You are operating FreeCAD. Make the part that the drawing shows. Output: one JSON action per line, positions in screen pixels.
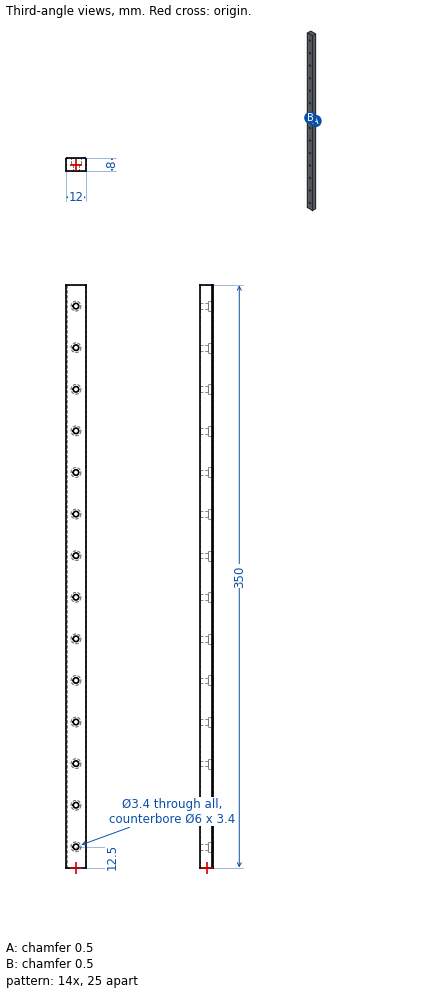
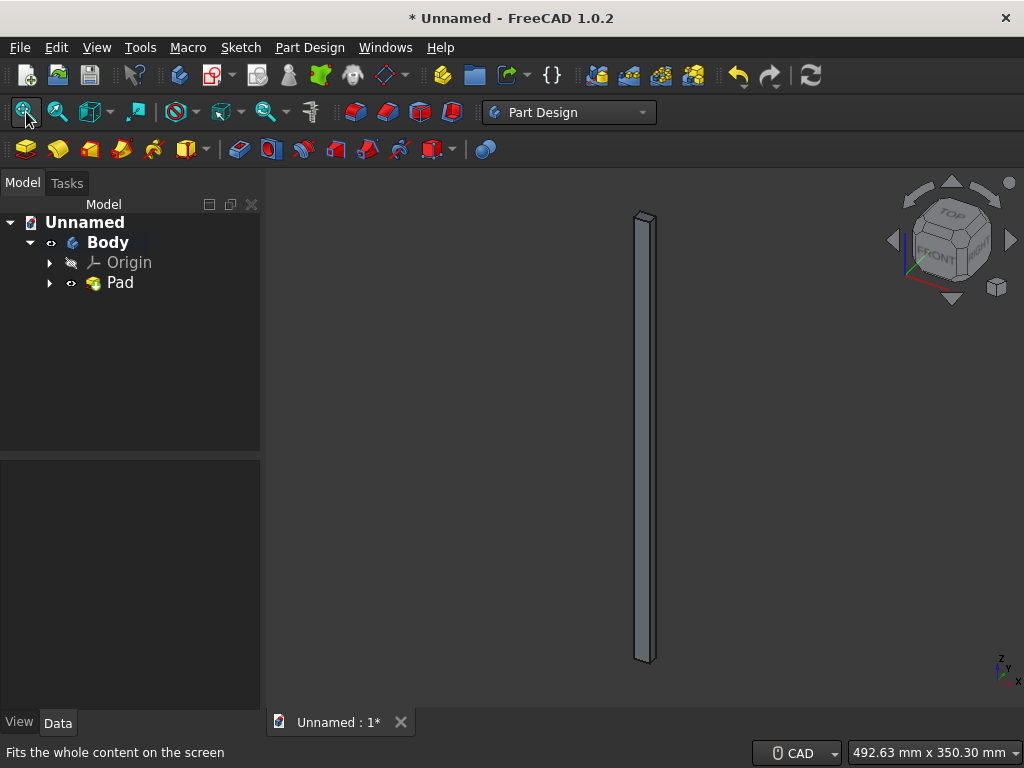
{"action": "key", "text": "0"}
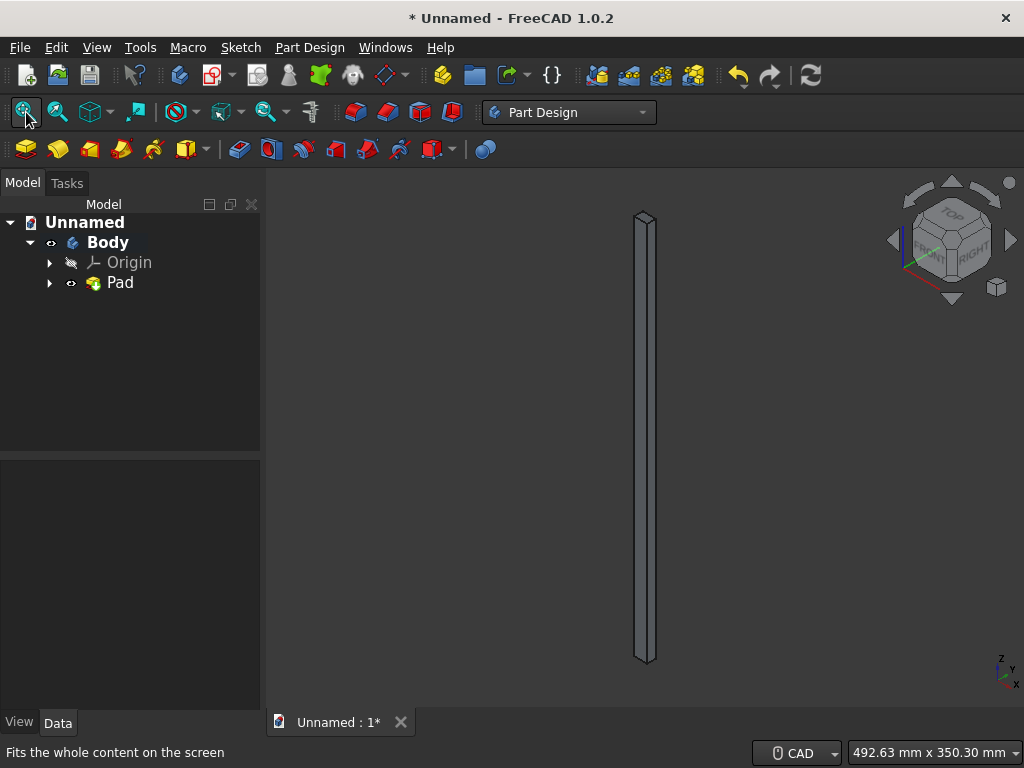
{"action": "key", "text": "2"}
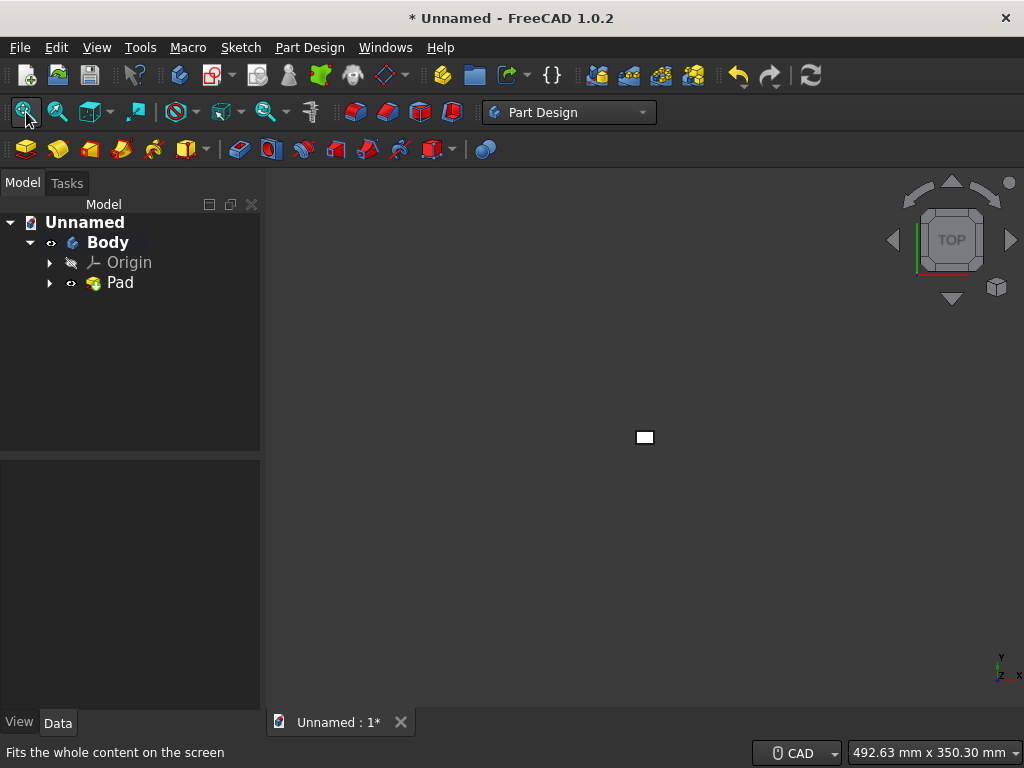
{"action": "left_click", "coordinate": [26, 112]}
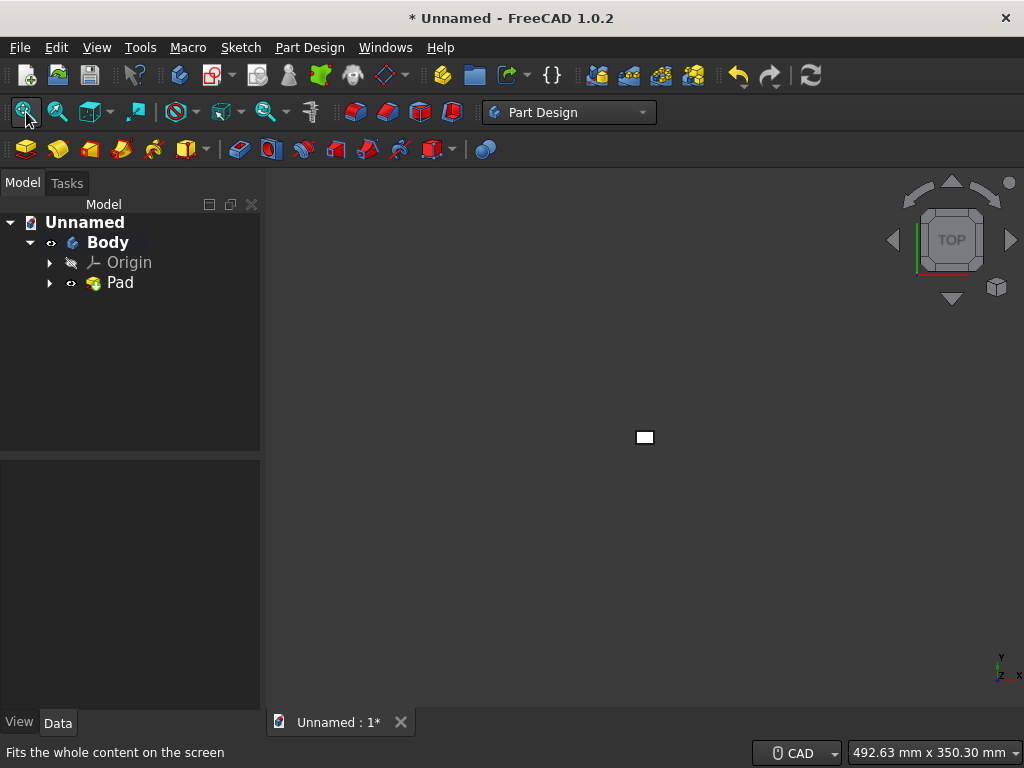
{"action": "key", "text": "1"}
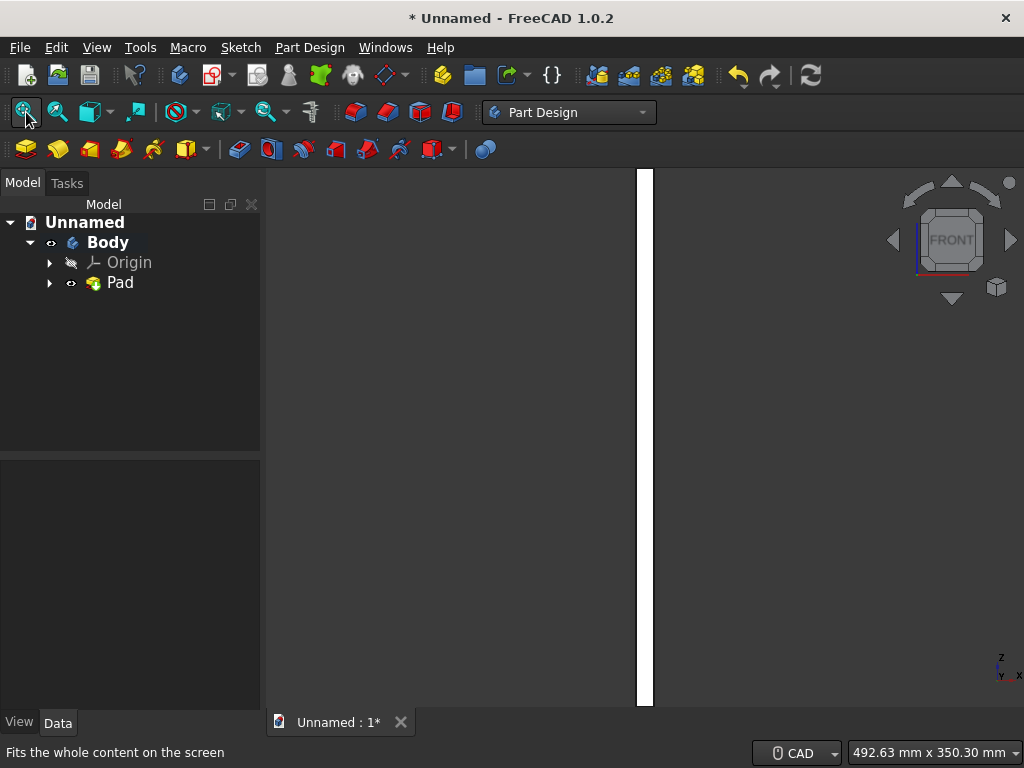
{"action": "left_click", "coordinate": [26, 112]}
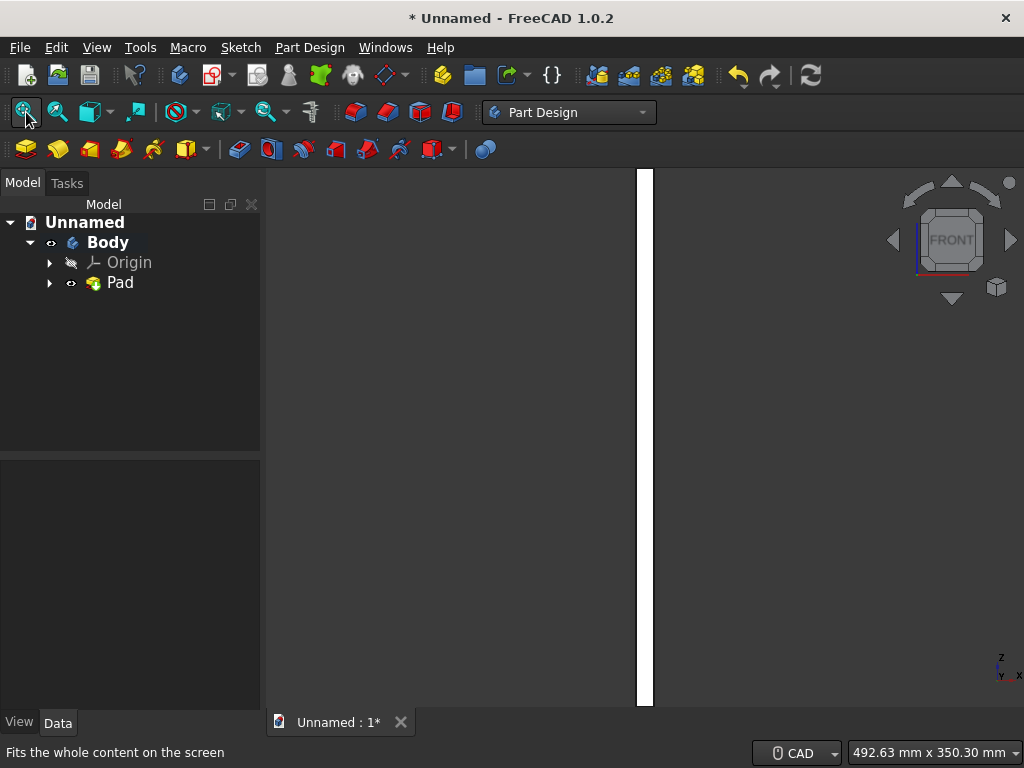
{"action": "key", "text": "3"}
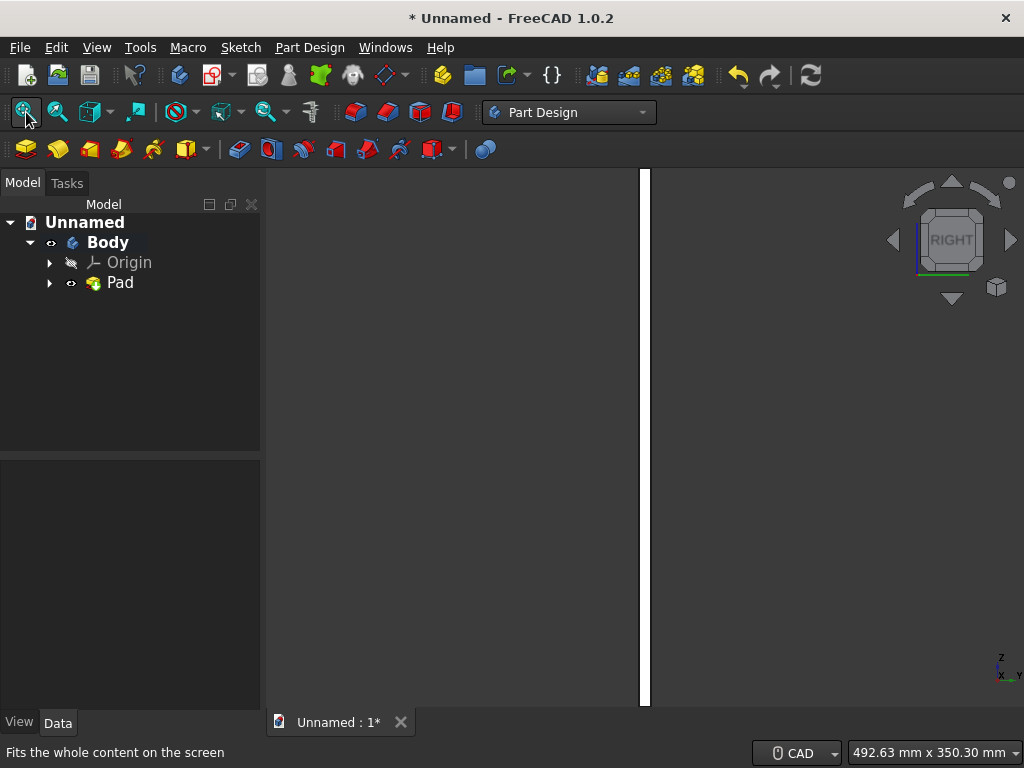
{"action": "left_click", "coordinate": [26, 112]}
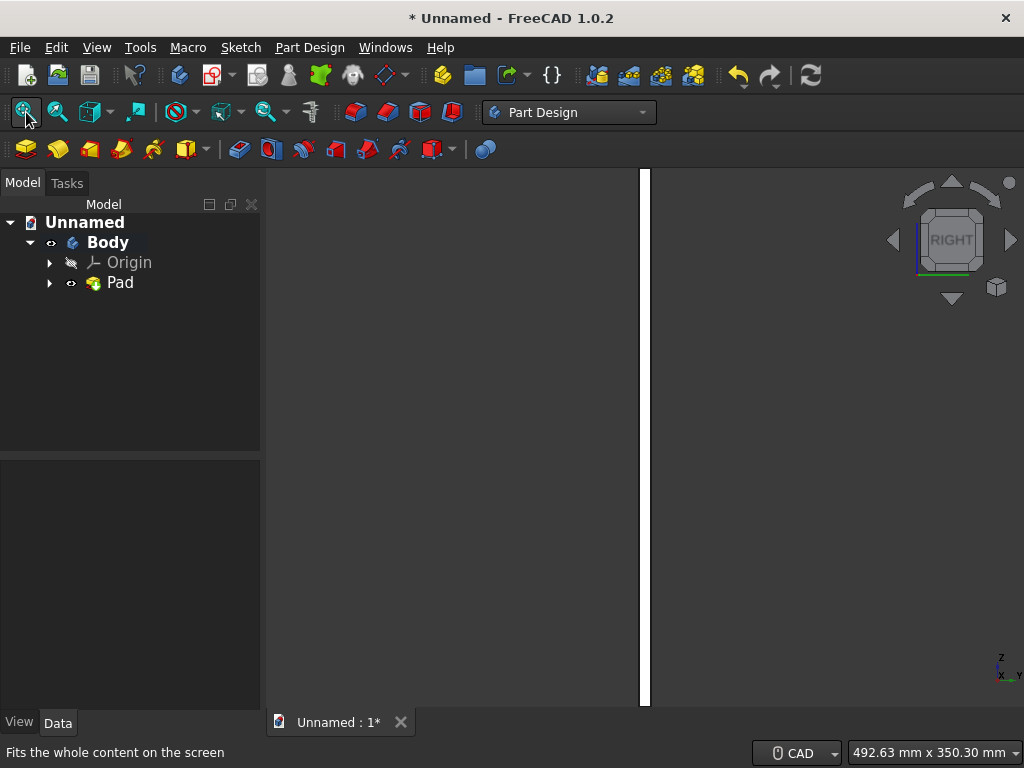
{"action": "left_click", "coordinate": [651, 436]}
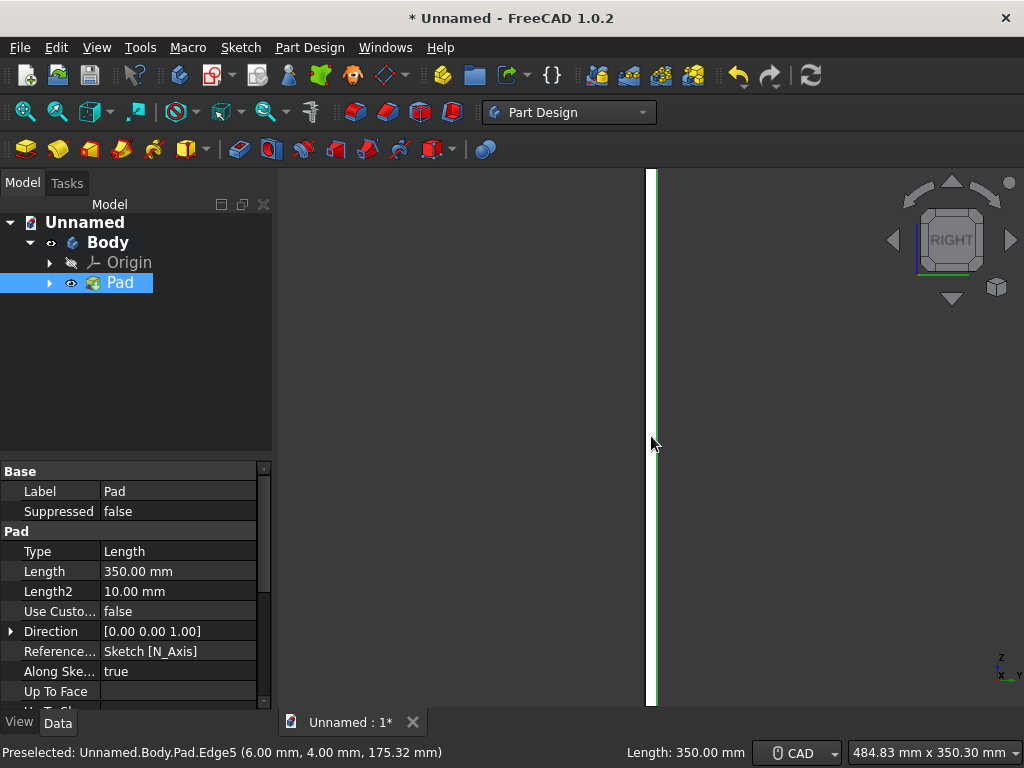
{"action": "left_click", "coordinate": [388, 112]}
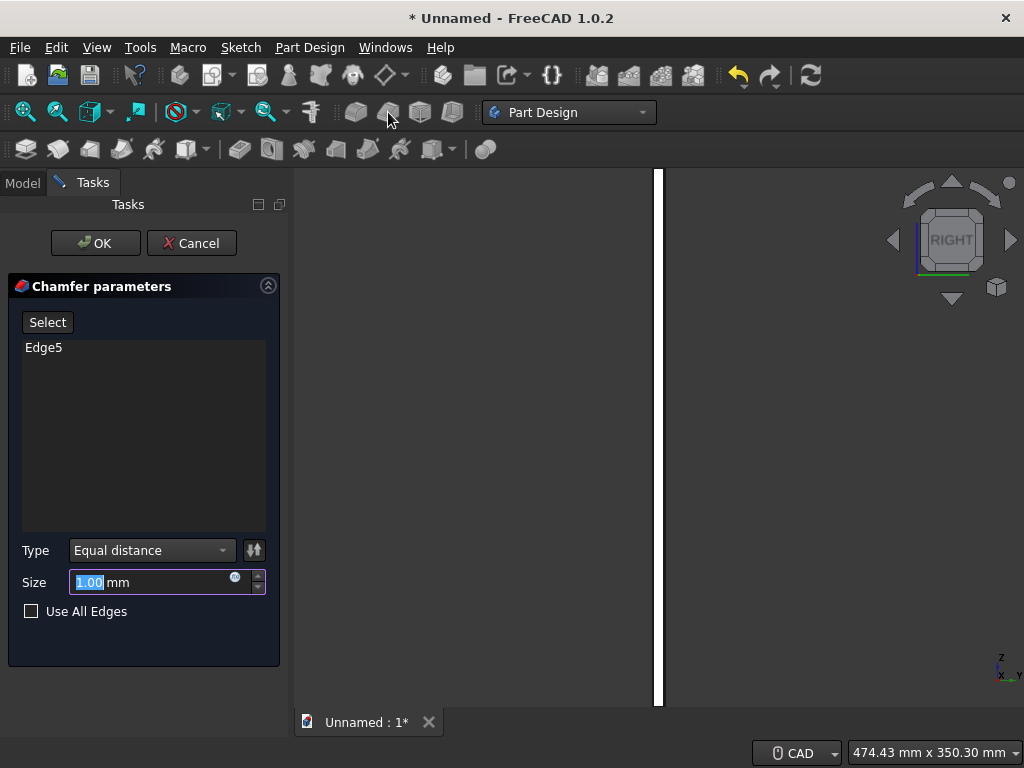
{"action": "type", "text": "0.5"}
{"action": "key", "text": "Tab"}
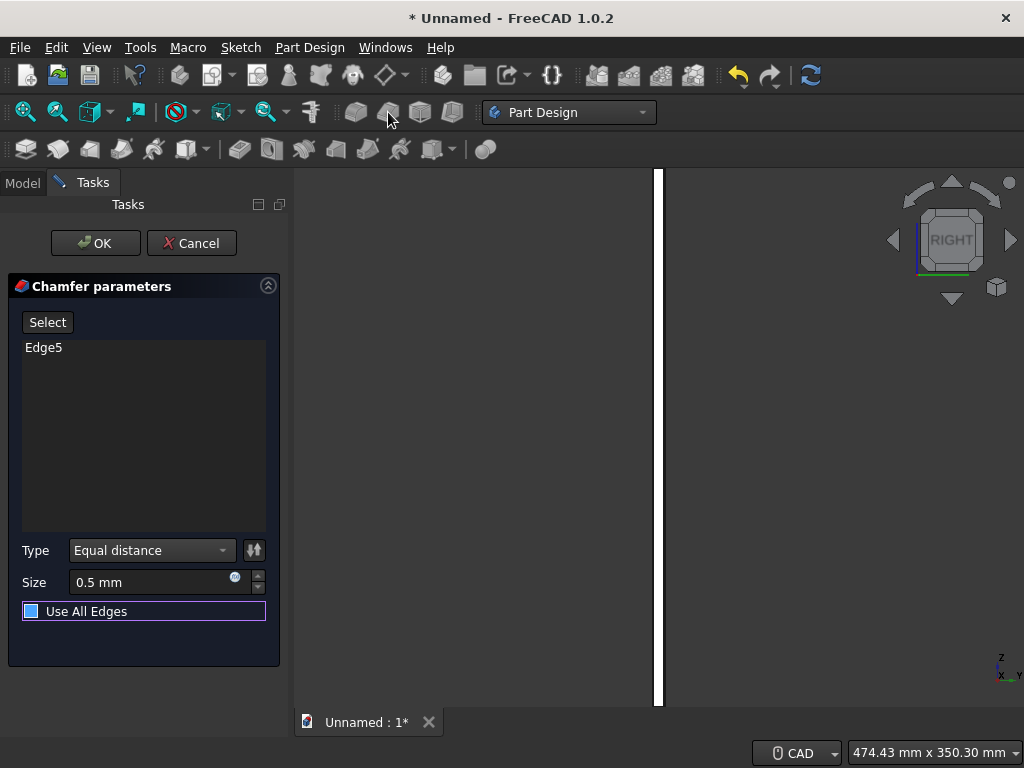
{"action": "left_click", "coordinate": [96, 243]}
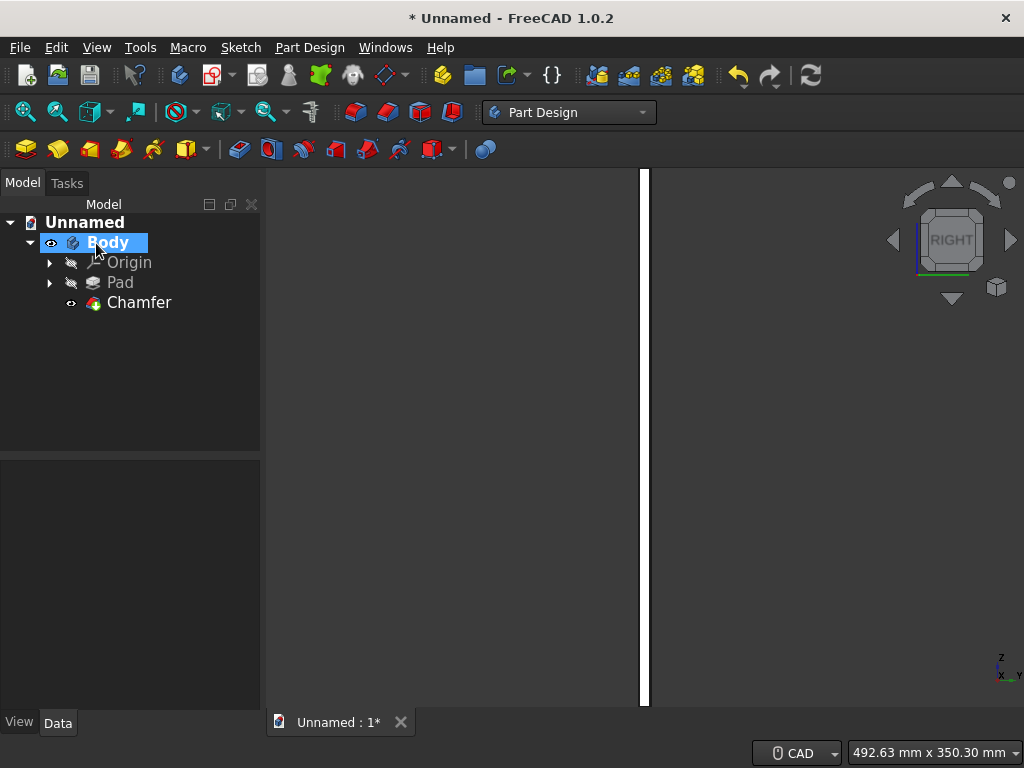
{"action": "left_click", "coordinate": [26, 112]}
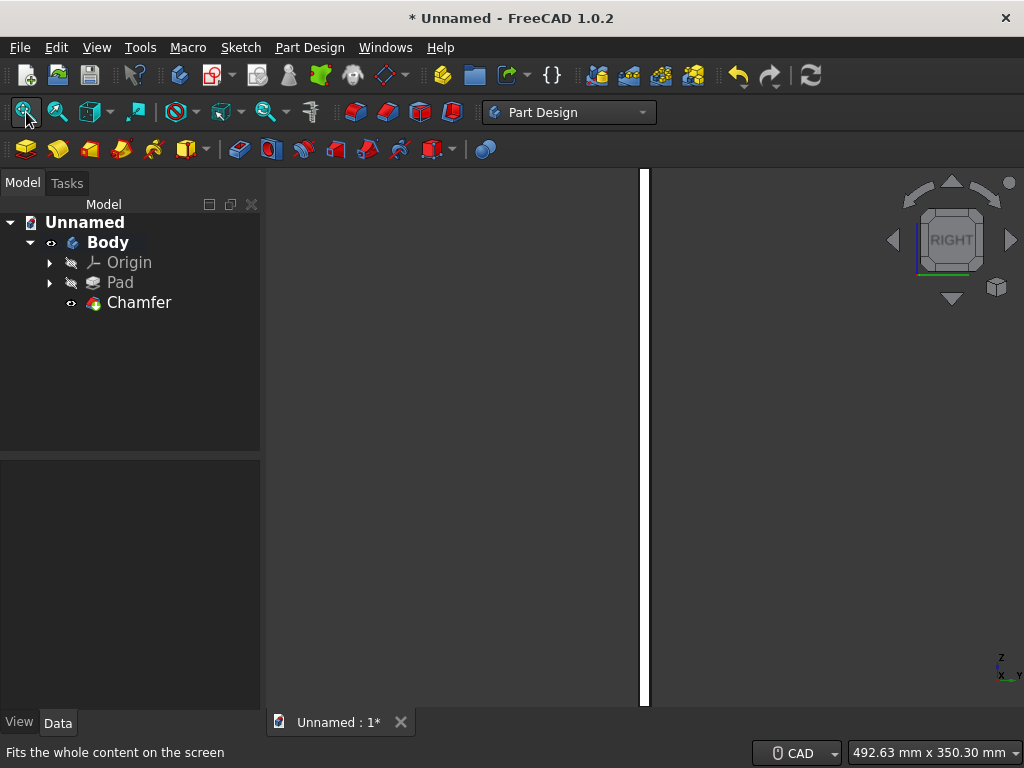
{"action": "key", "text": "0"}